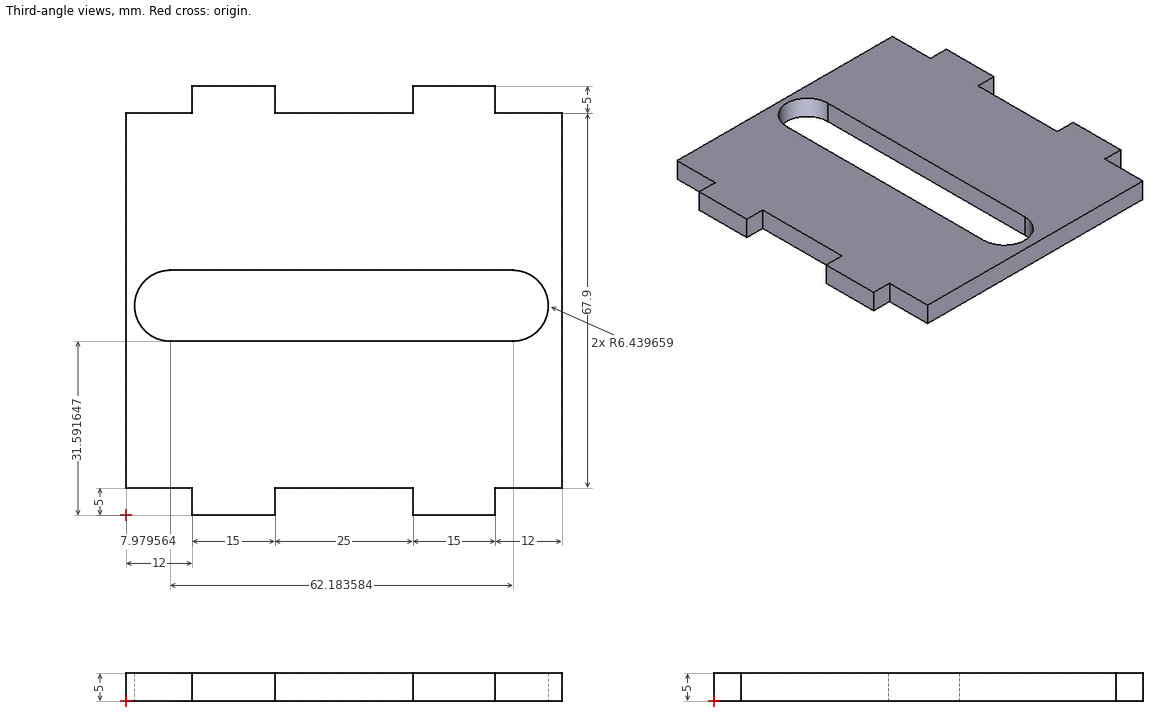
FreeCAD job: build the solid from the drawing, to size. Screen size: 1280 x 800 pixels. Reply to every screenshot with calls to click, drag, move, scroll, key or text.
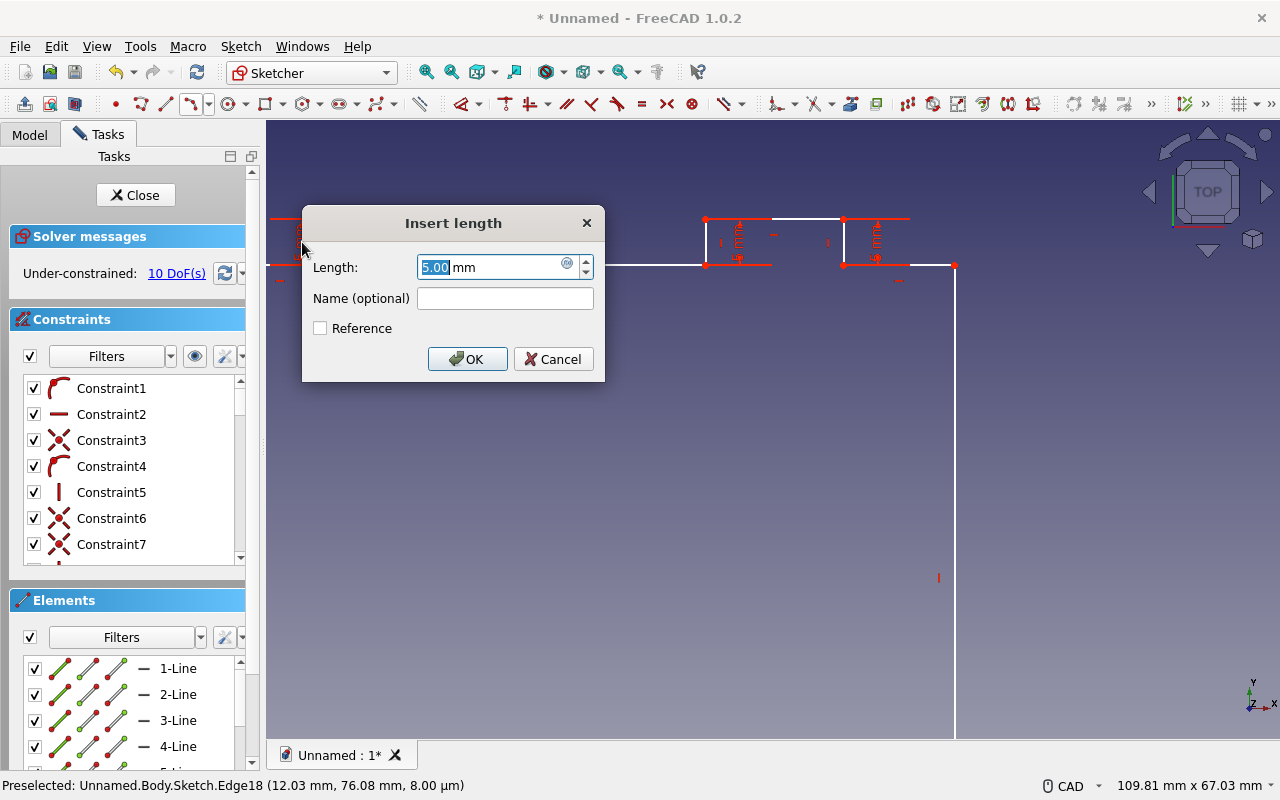
text(5)
key(Return)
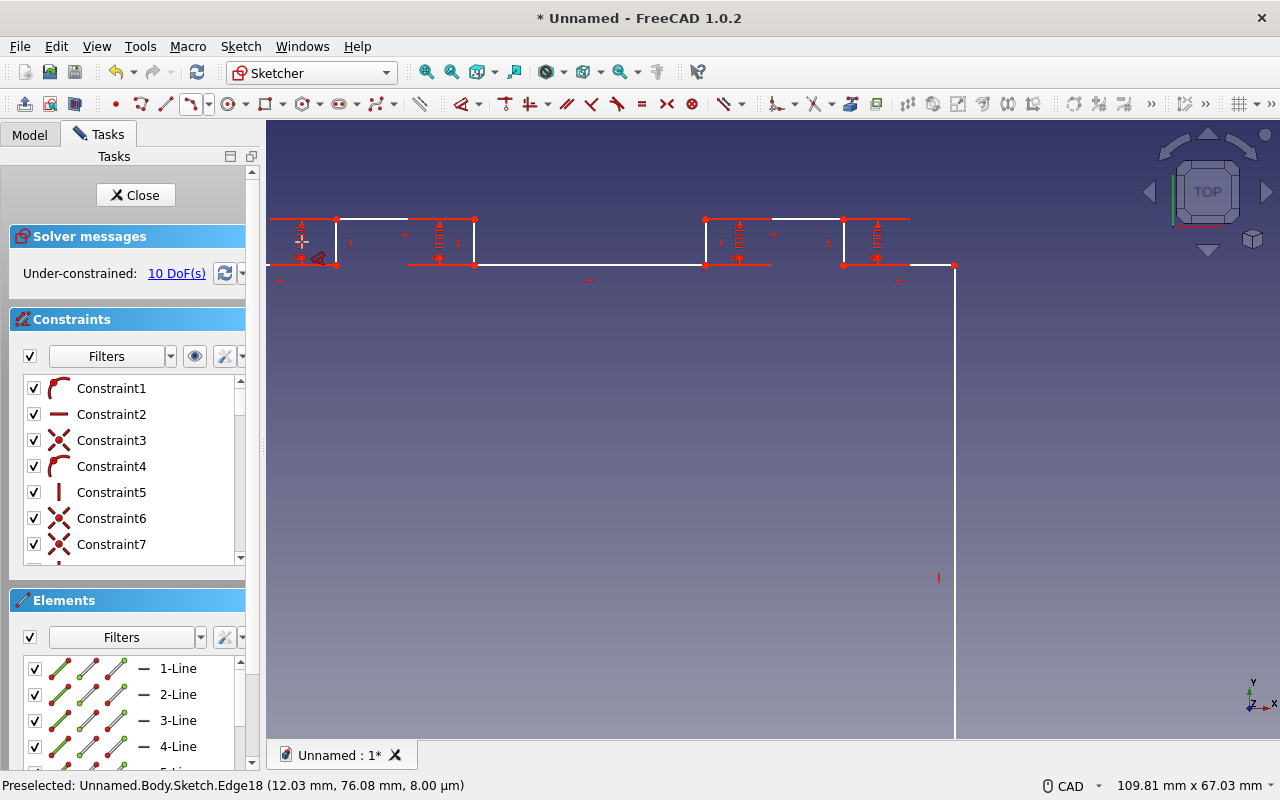
scroll(844, 250, down, 3)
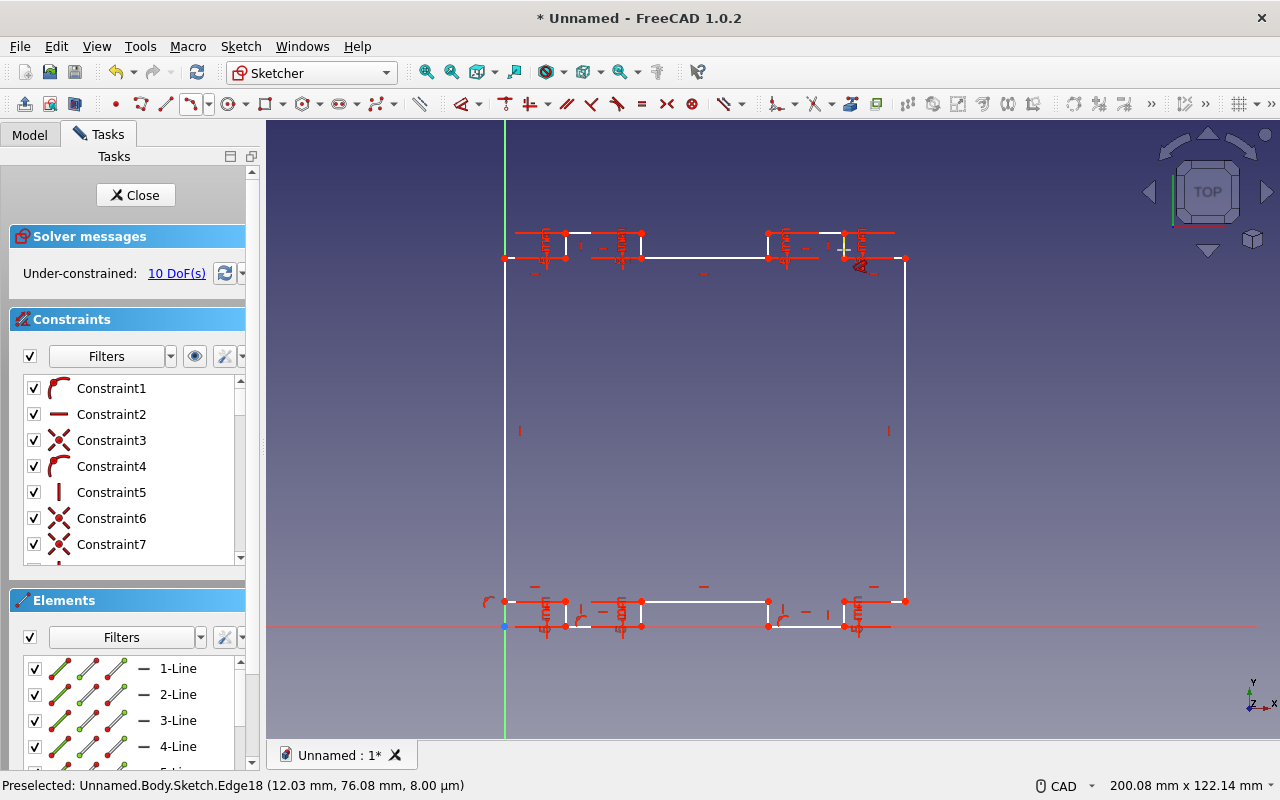
click(523, 602)
click(535, 568)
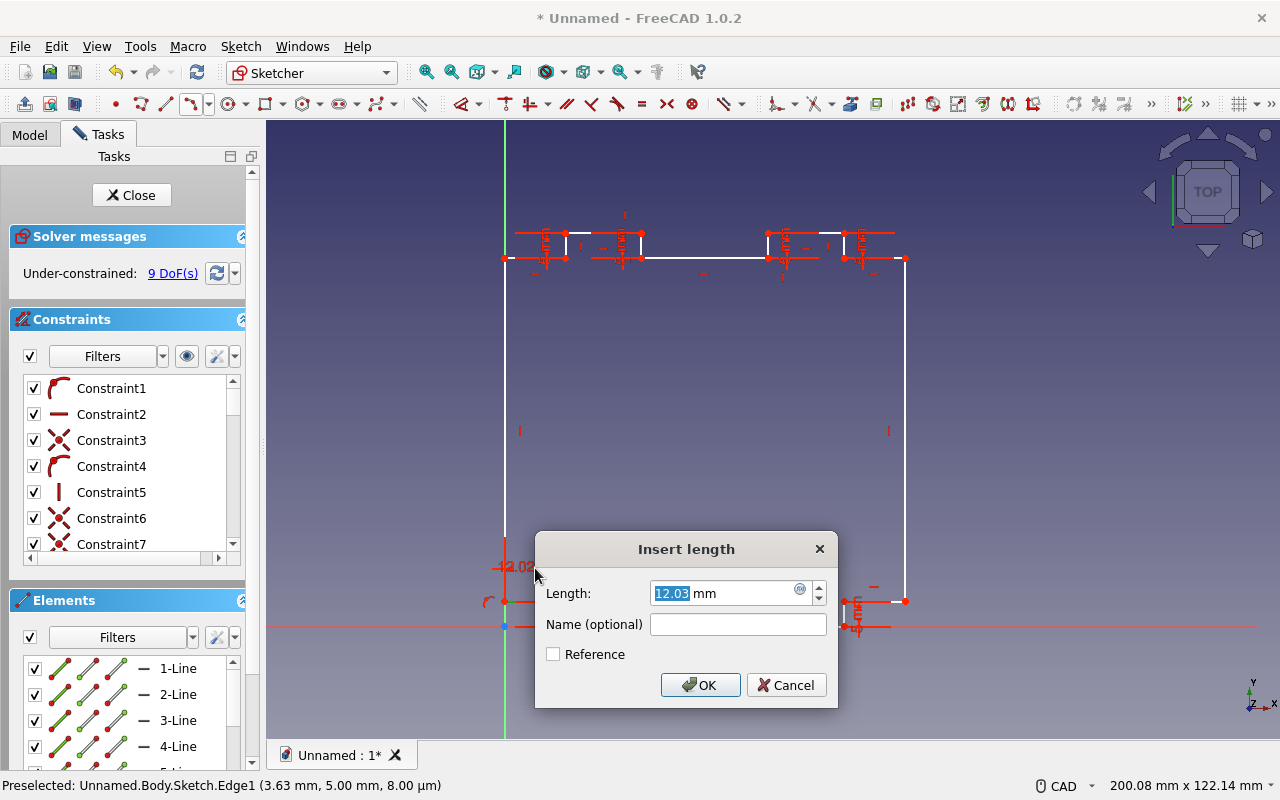
text(12)
key(Return)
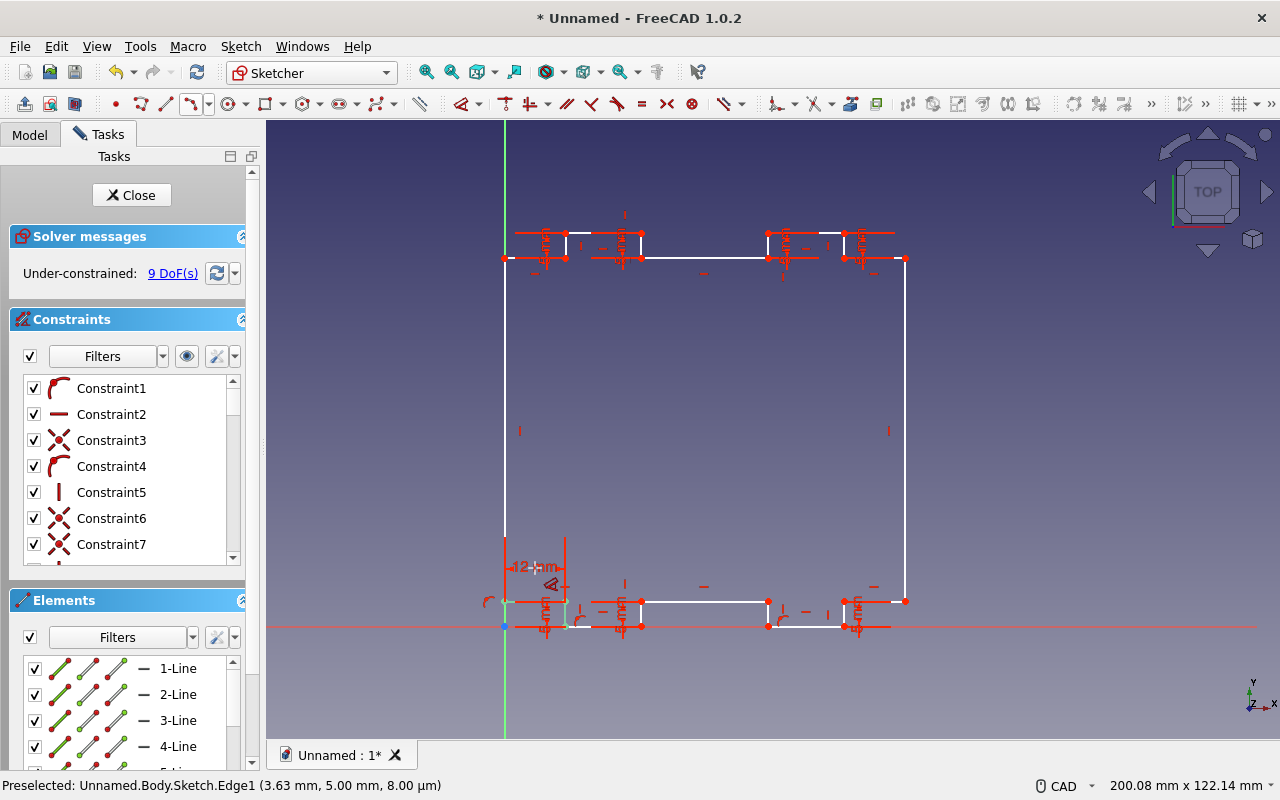
click(588, 627)
click(603, 661)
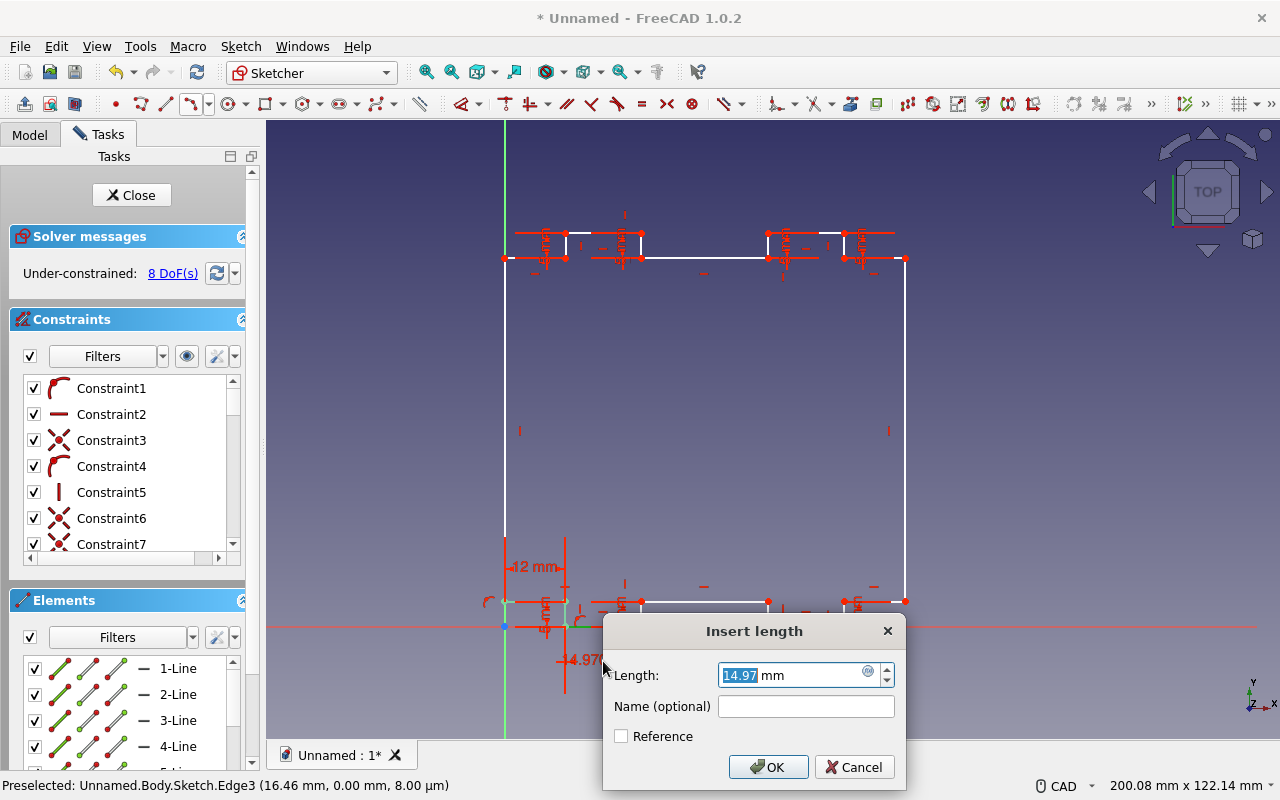
text(15)
key(Return)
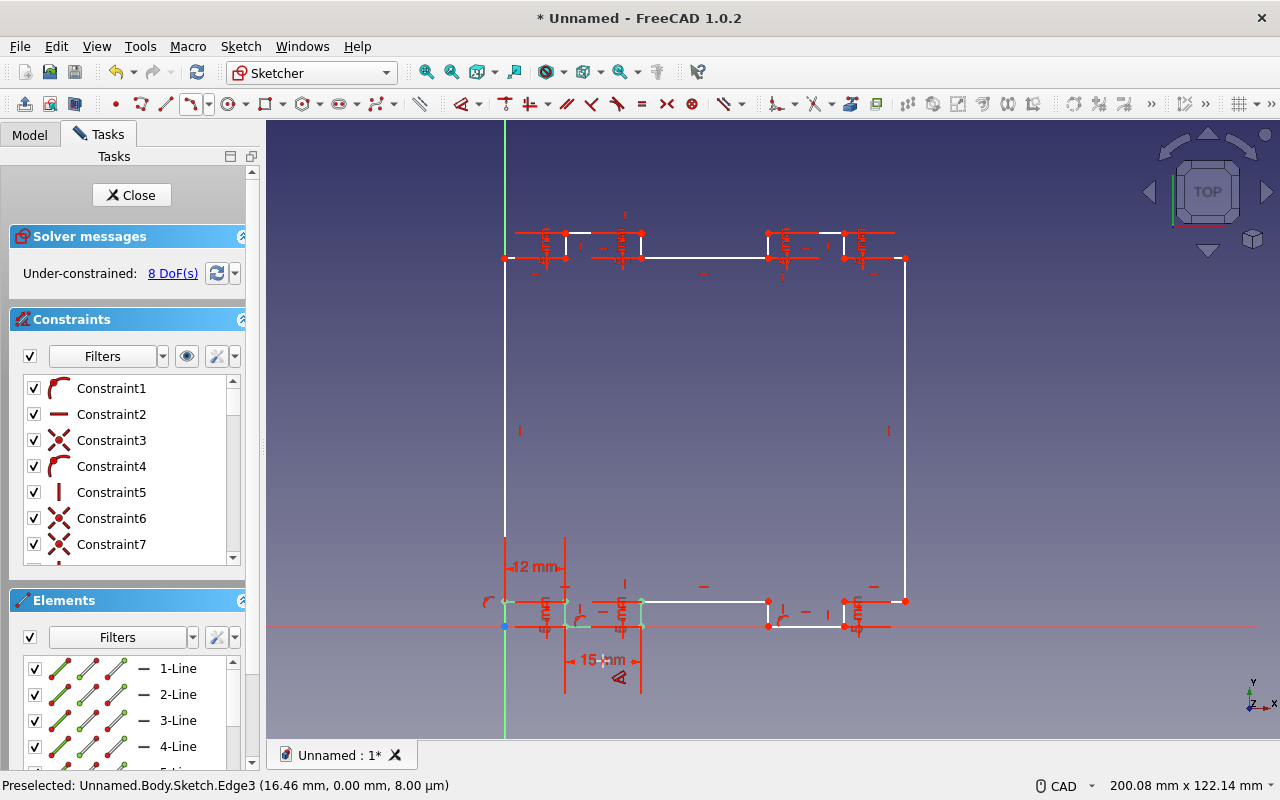
click(679, 602)
click(705, 568)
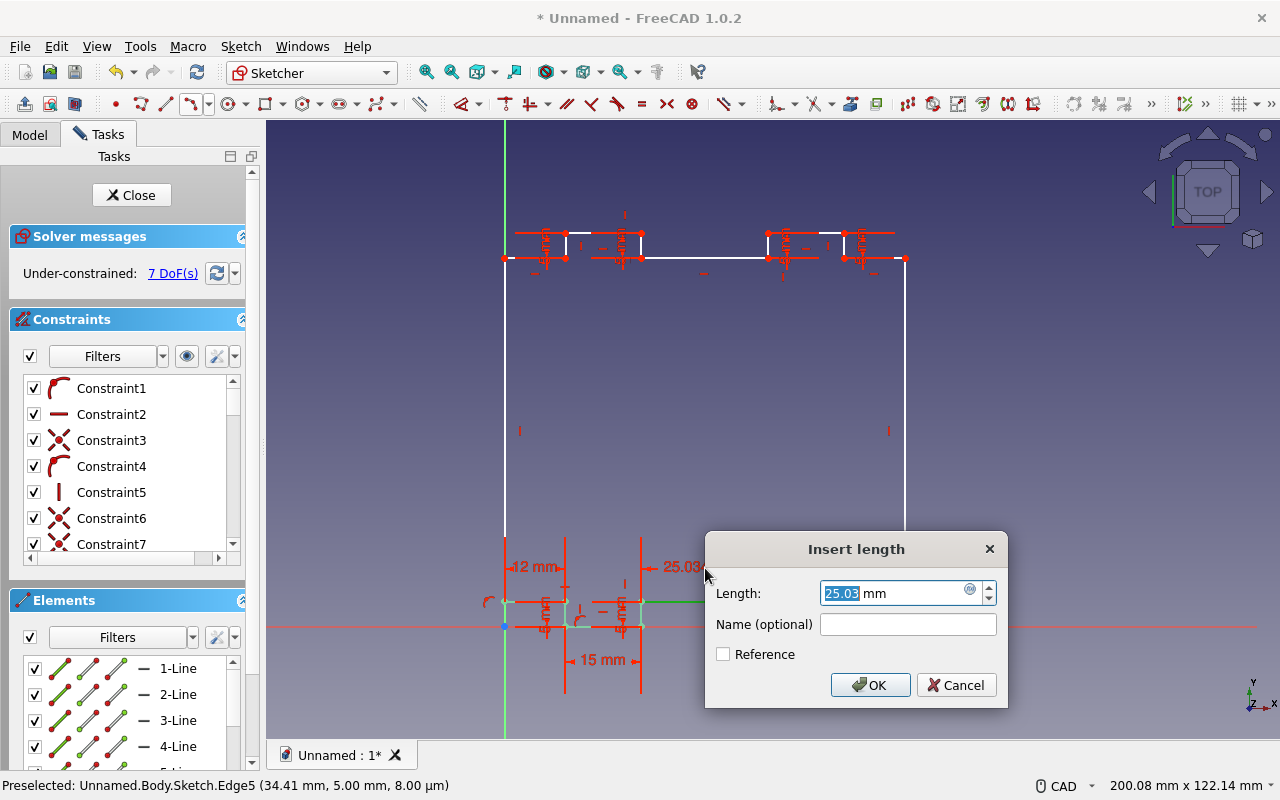
text(25)
key(Return)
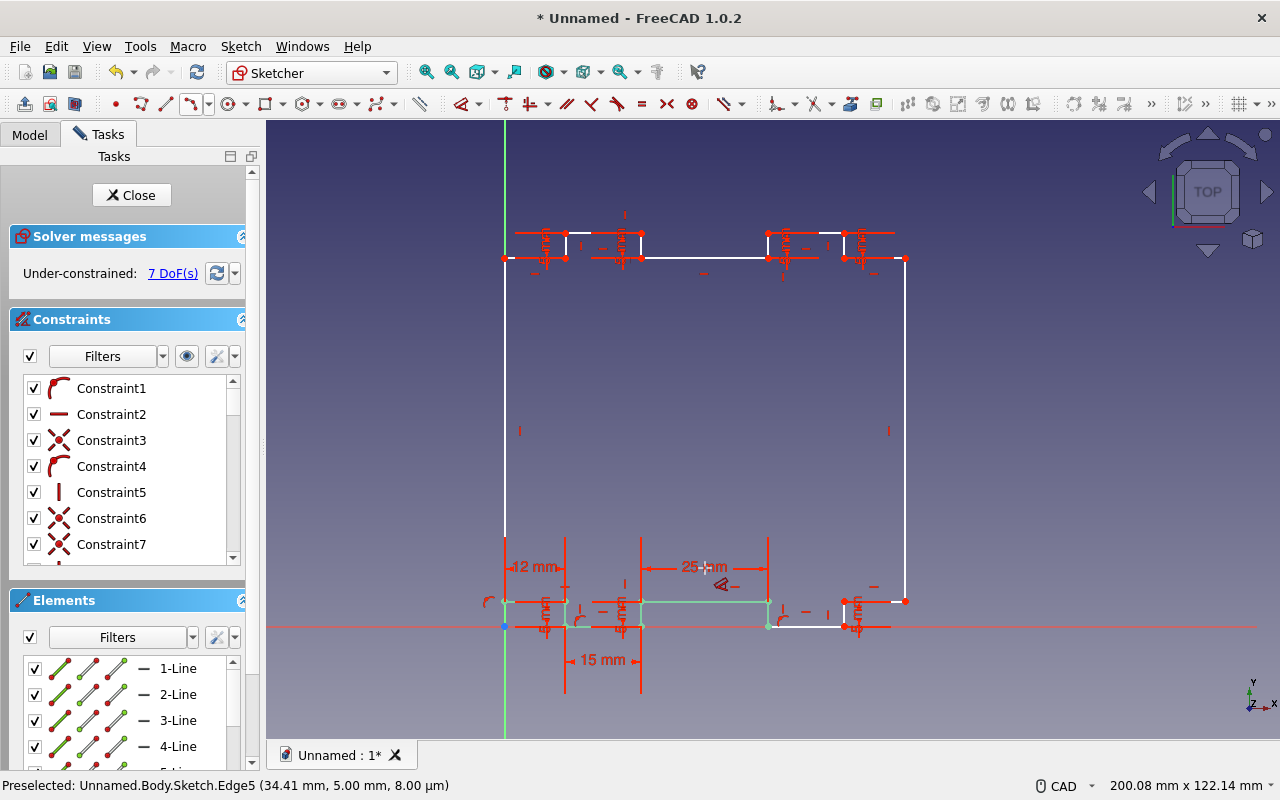
click(791, 627)
click(806, 661)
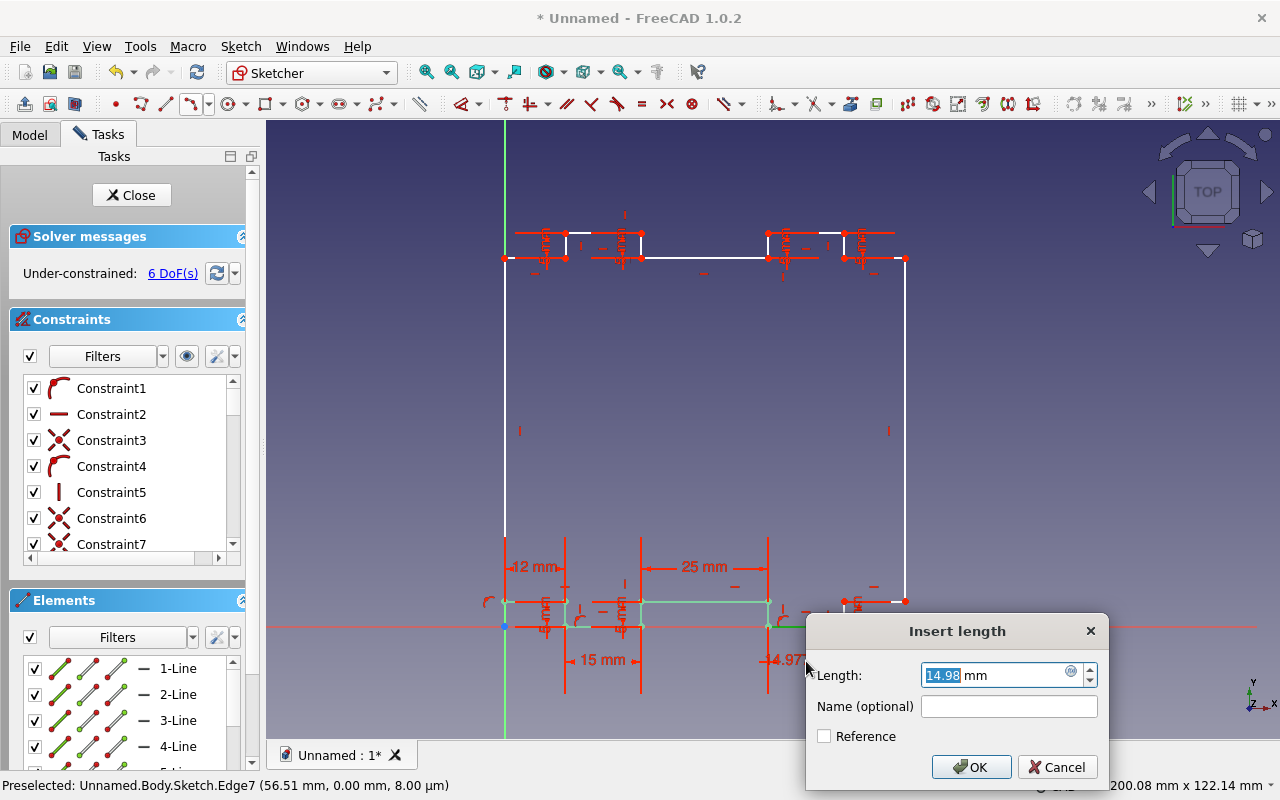
text(15)
key(Return)